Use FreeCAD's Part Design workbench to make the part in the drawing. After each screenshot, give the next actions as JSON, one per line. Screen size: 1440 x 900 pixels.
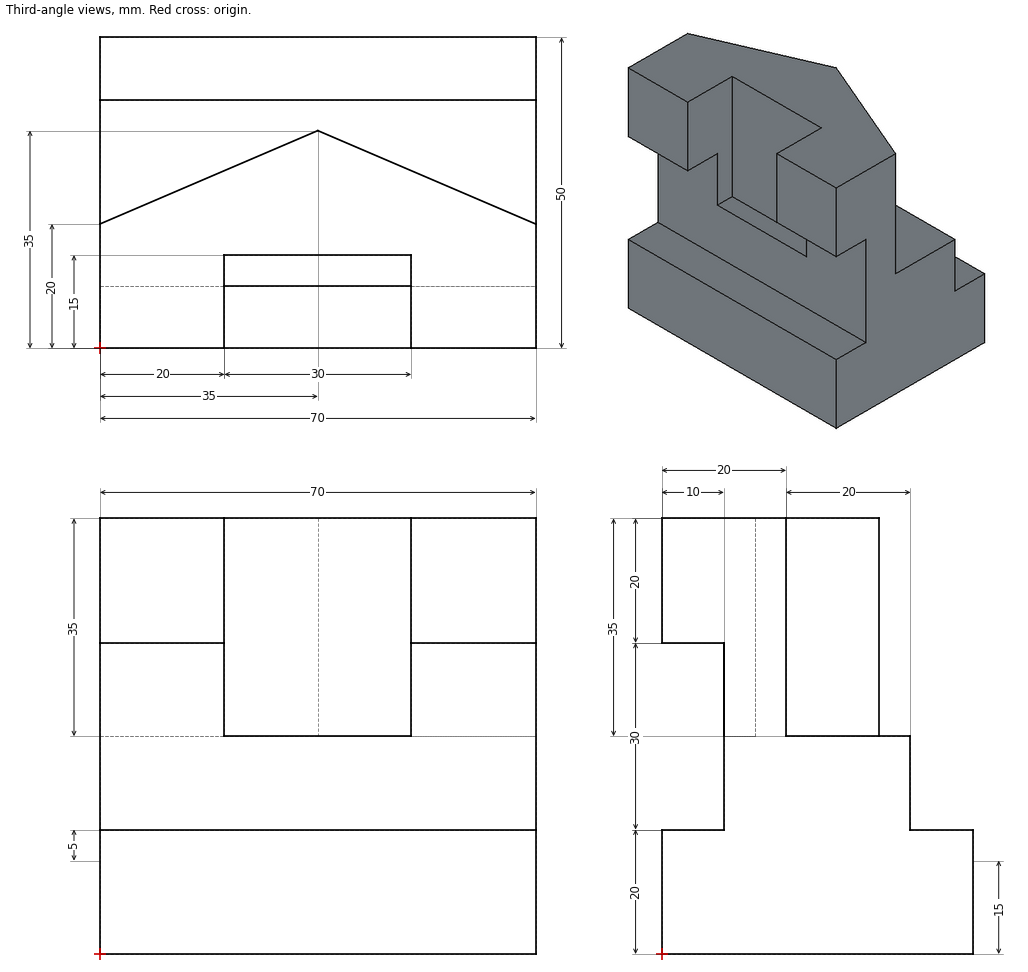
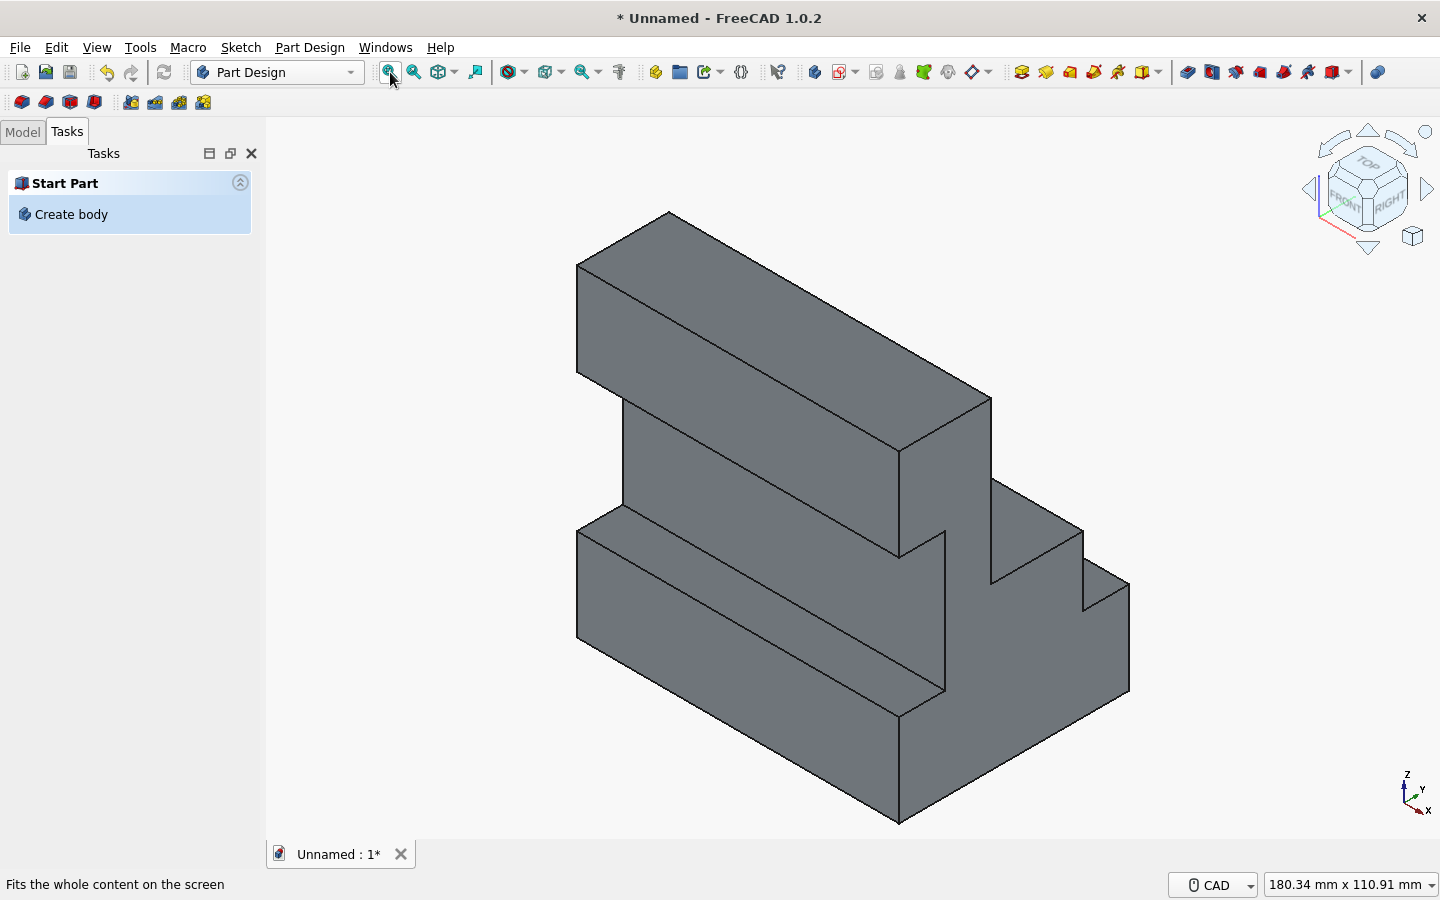
{"action": "left_click", "coordinate": [876, 384]}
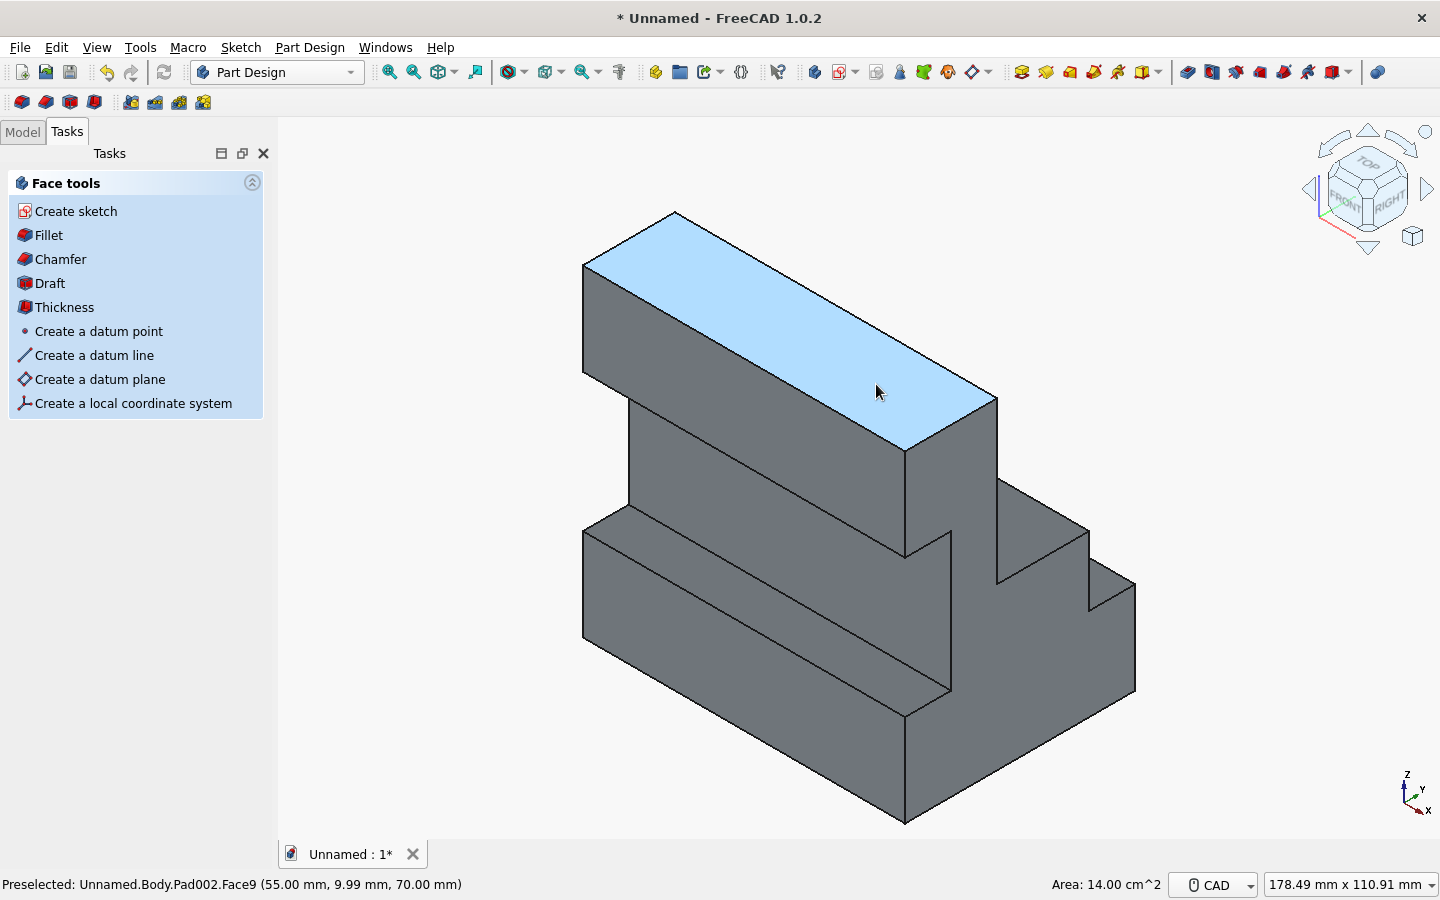
{"action": "left_click", "coordinate": [840, 72]}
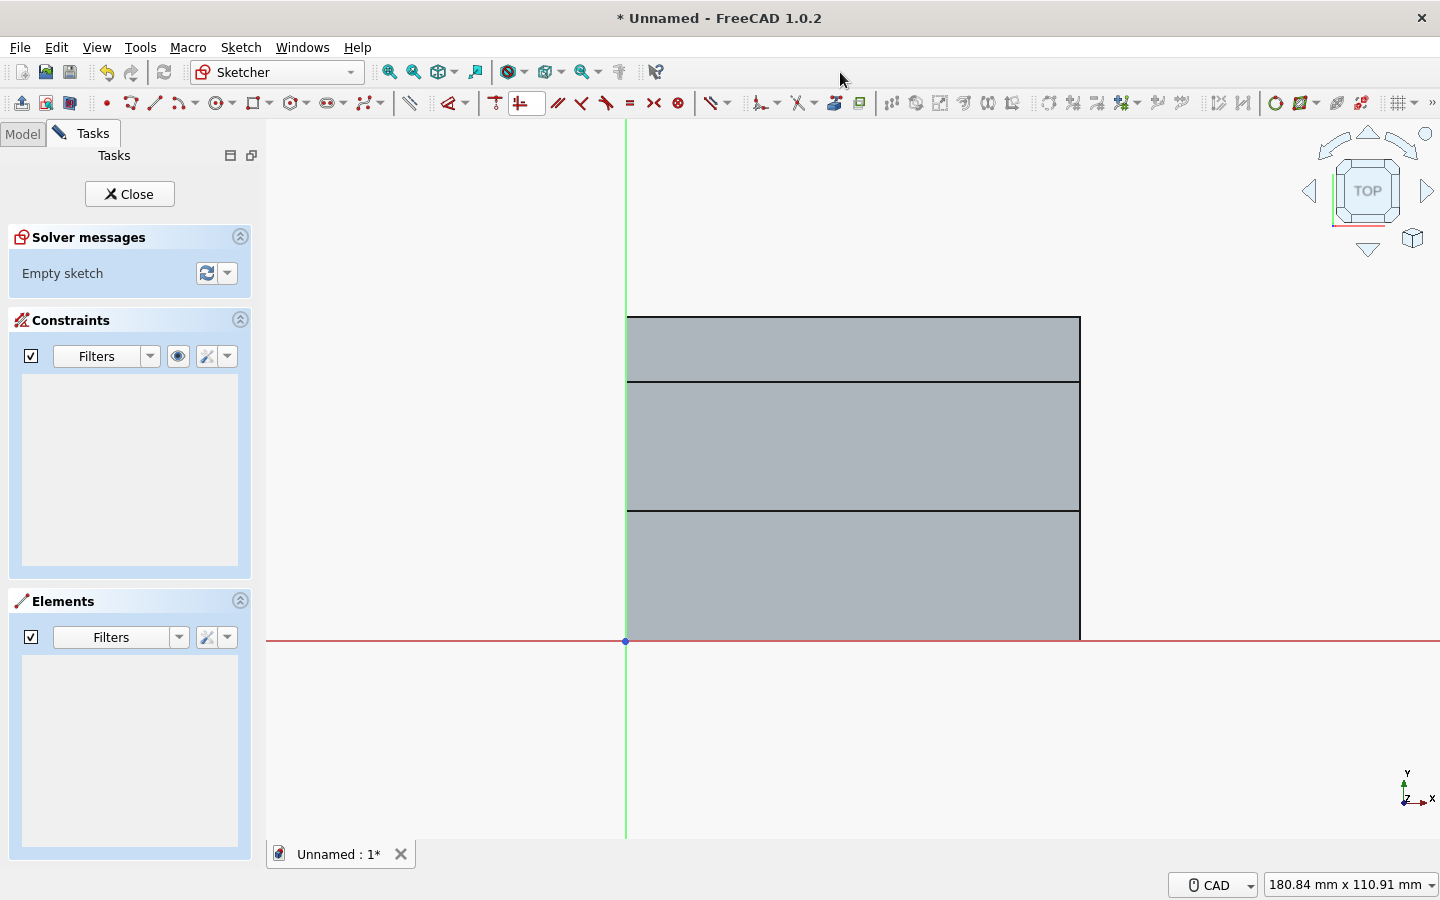
{"action": "scroll", "coordinate": [992, 627], "scroll_direction": "up", "scroll_amount": 2}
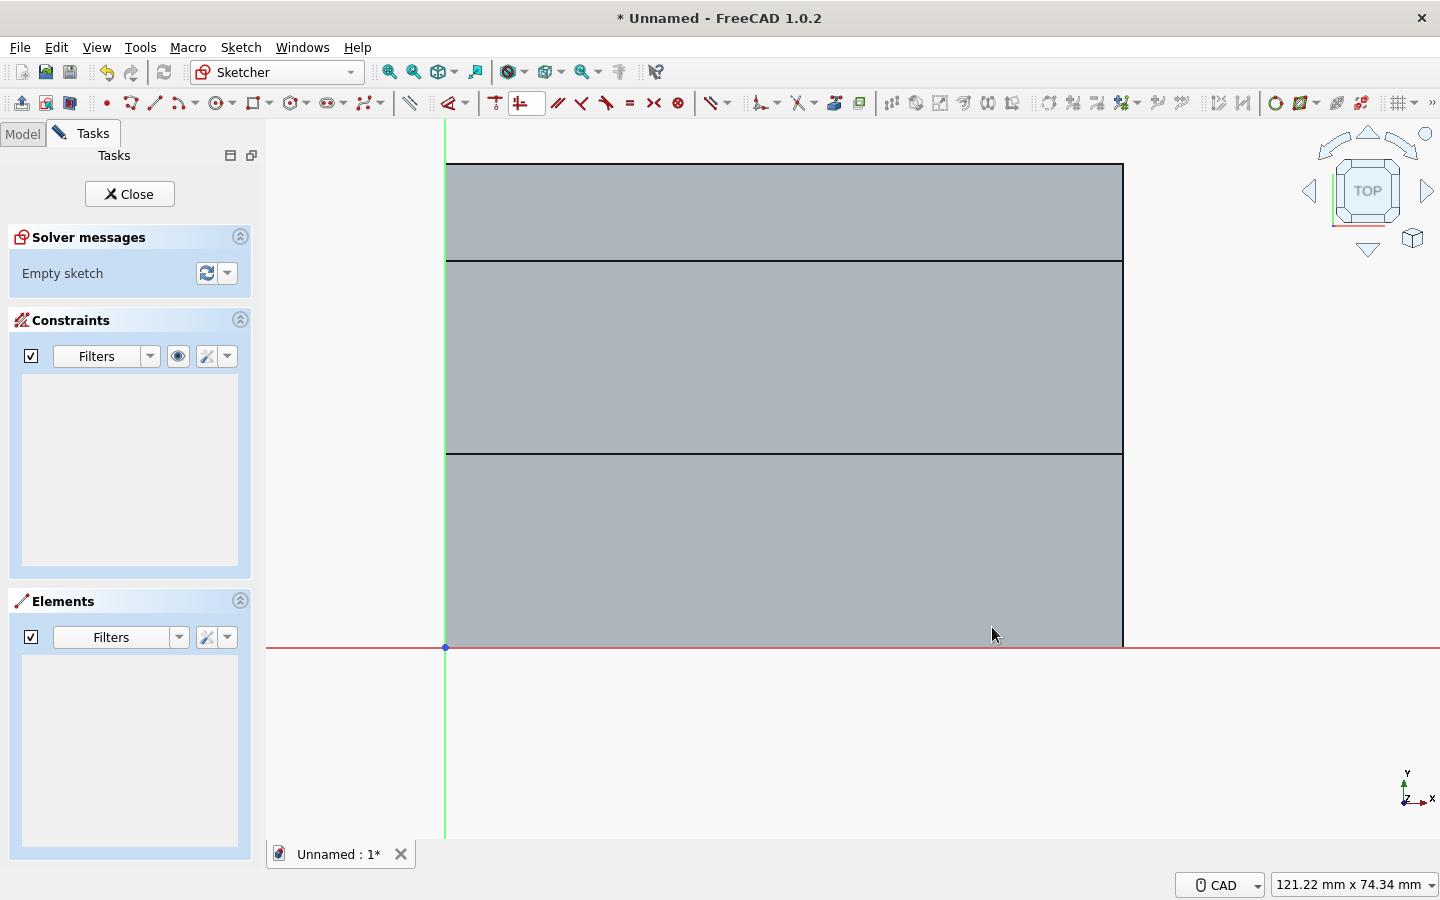
{"action": "left_click", "coordinate": [132, 104]}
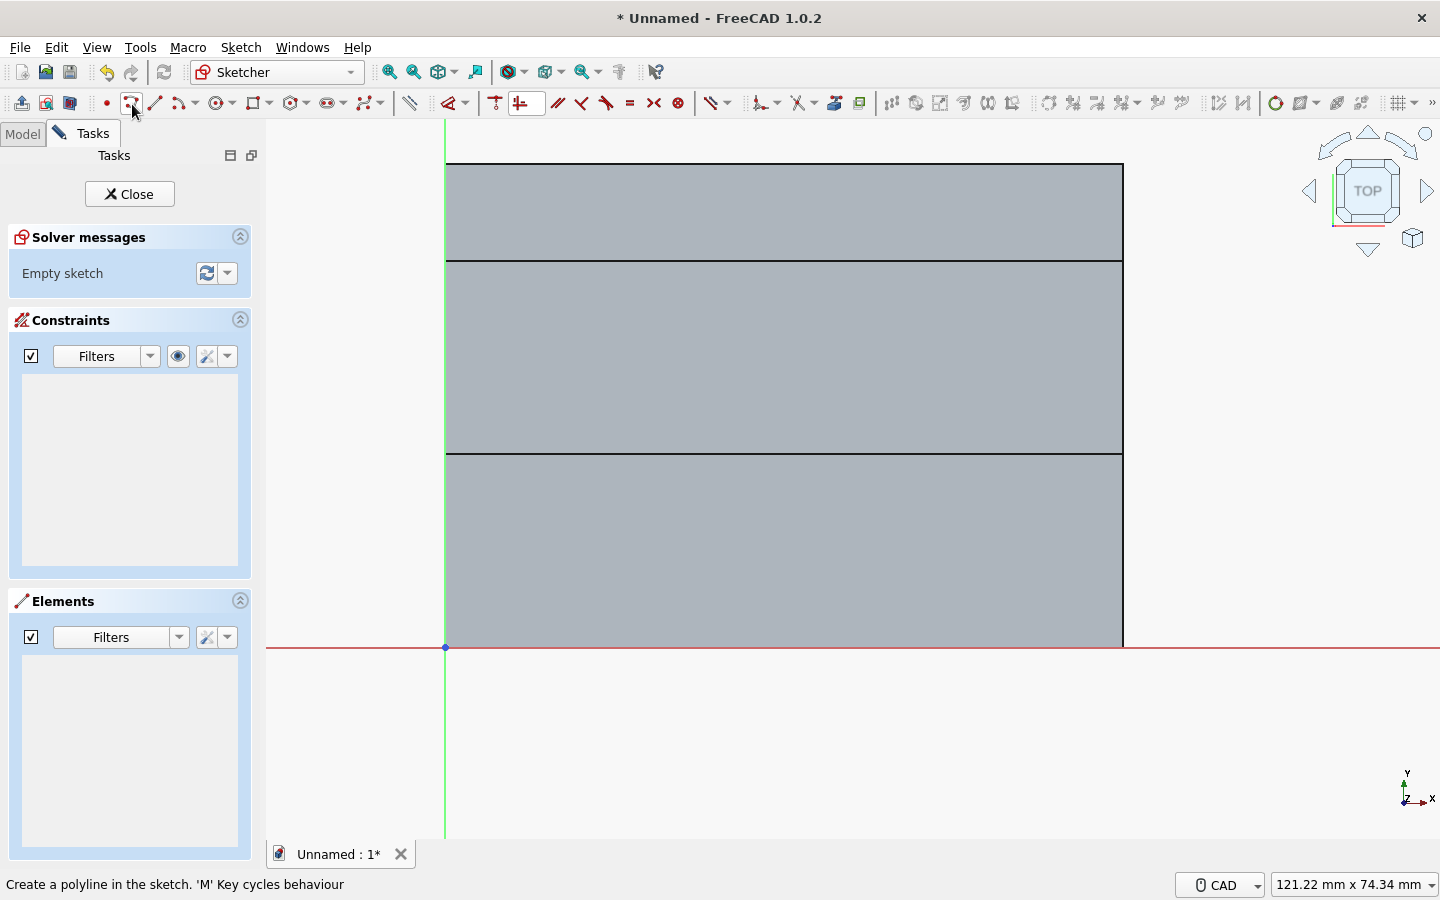
{"action": "left_click", "coordinate": [445, 454]}
{"action": "left_click", "coordinate": [1123, 454]}
{"action": "left_click", "coordinate": [784, 309]}
{"action": "left_click", "coordinate": [445, 455]}
{"action": "key", "text": "Escape"}
{"action": "key", "text": "Escape"}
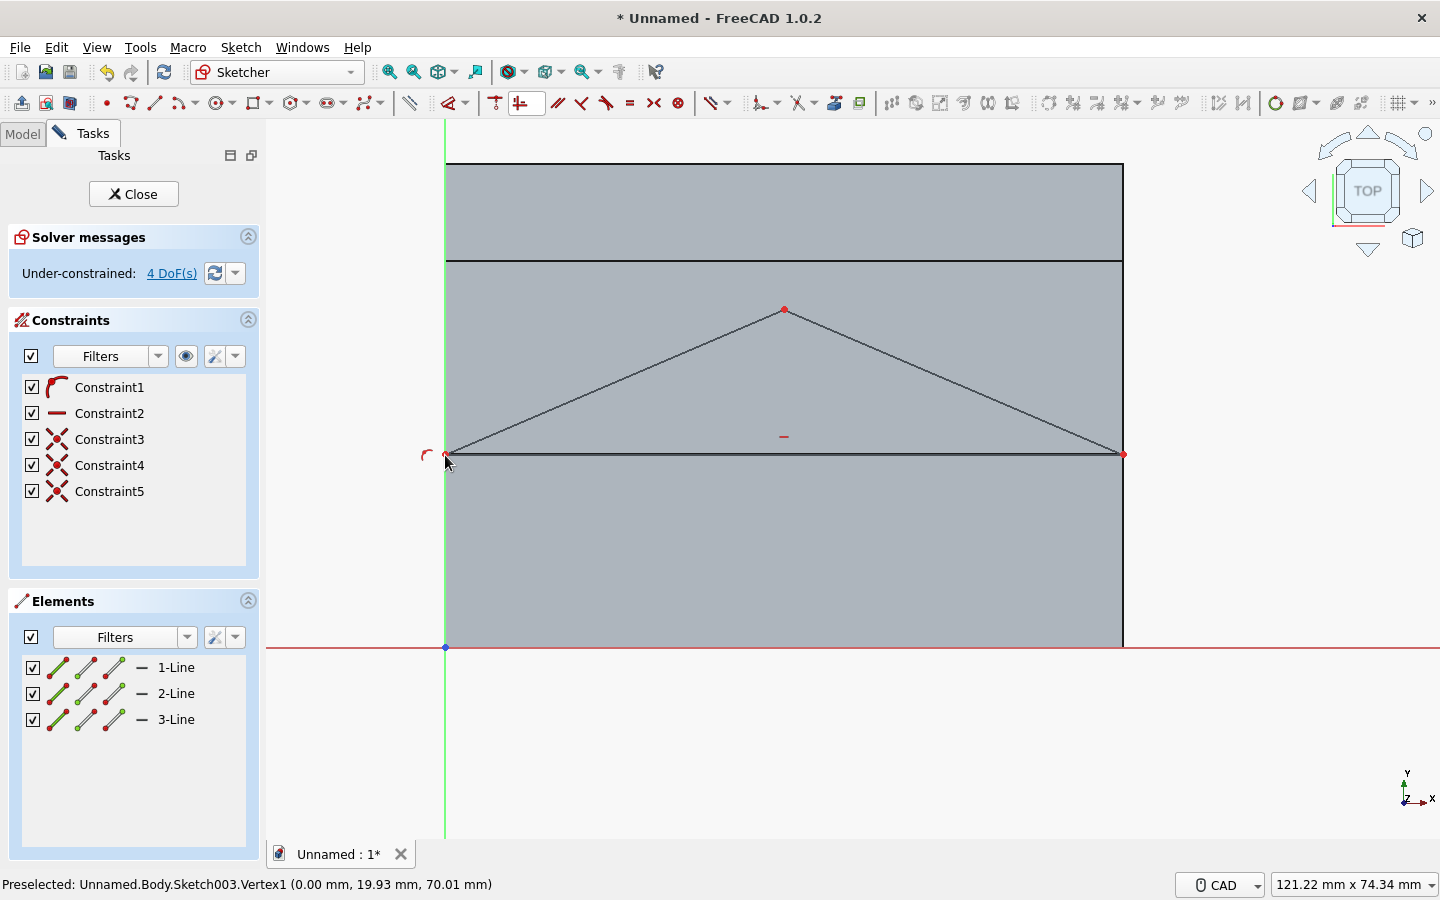
{"action": "left_click", "coordinate": [448, 104]}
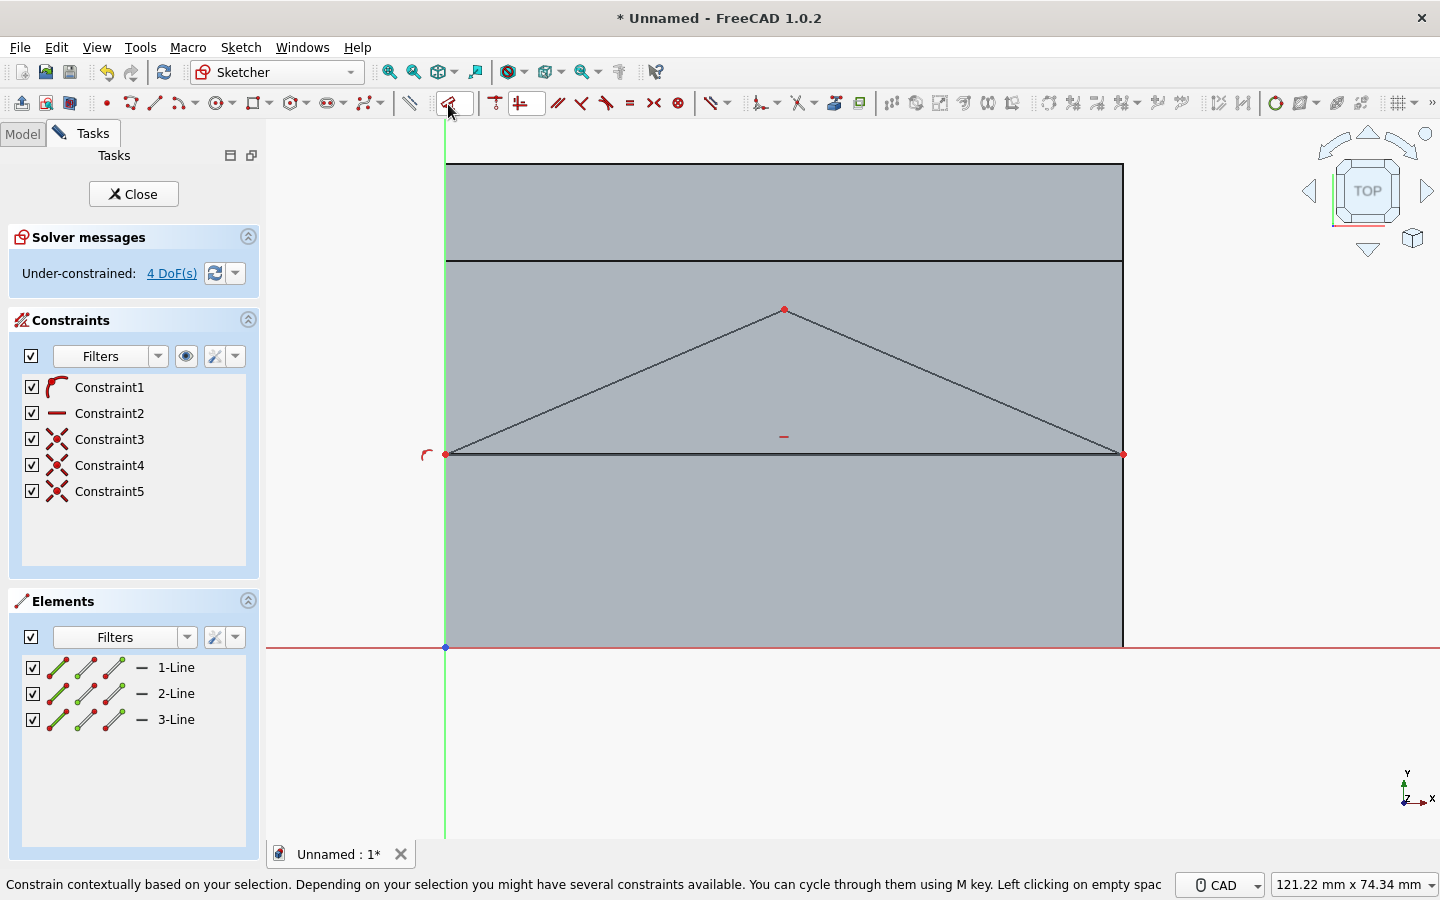
{"action": "left_click", "coordinate": [649, 455]}
{"action": "left_click", "coordinate": [784, 421]}